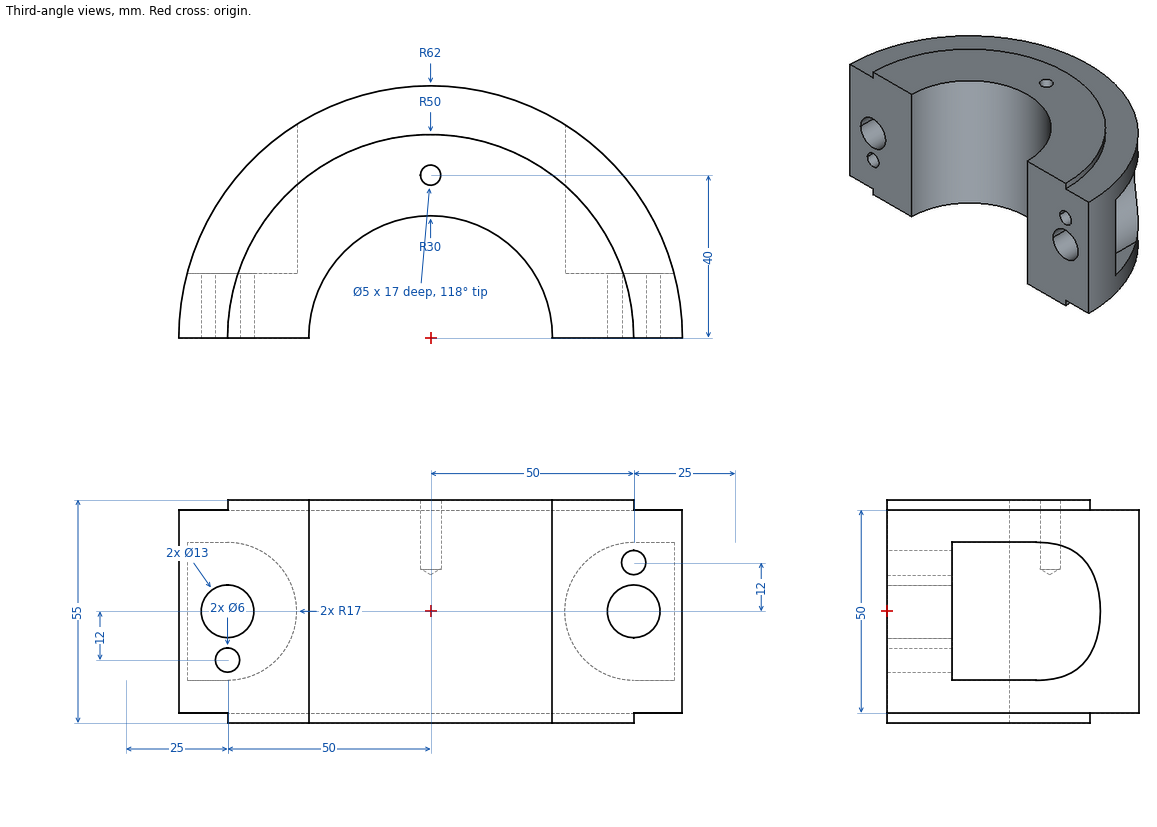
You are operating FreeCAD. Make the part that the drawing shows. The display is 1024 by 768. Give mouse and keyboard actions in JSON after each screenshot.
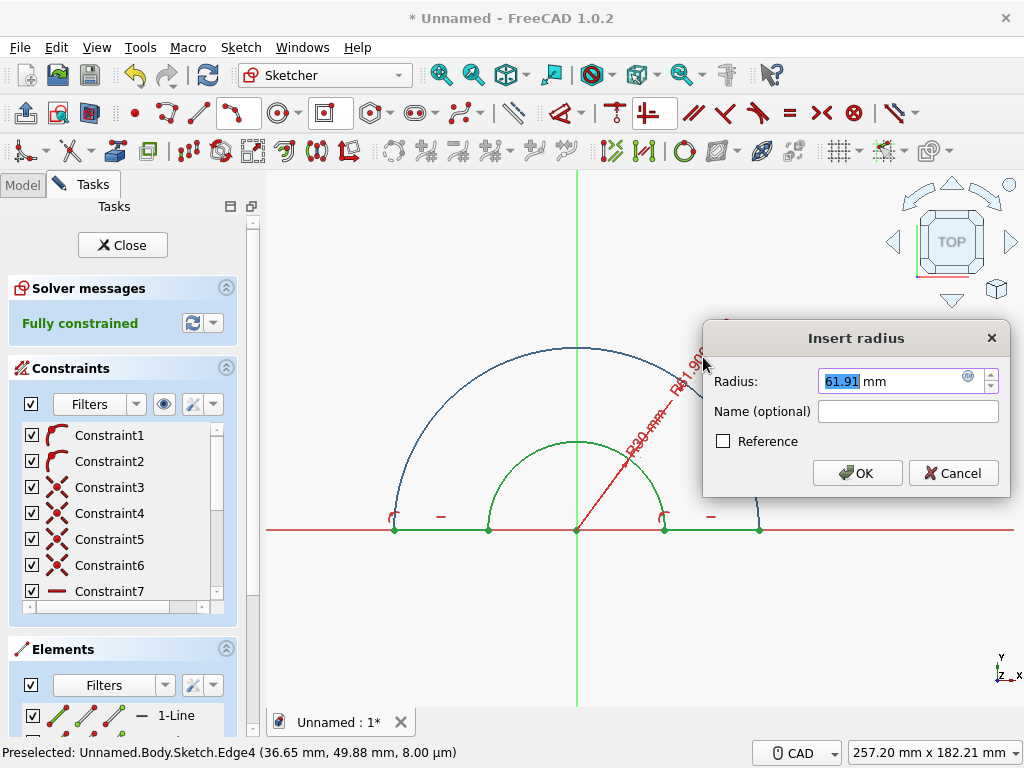
{"action": "type", "text": "62"}
{"action": "key", "text": "Return"}
{"action": "key", "text": "Escape"}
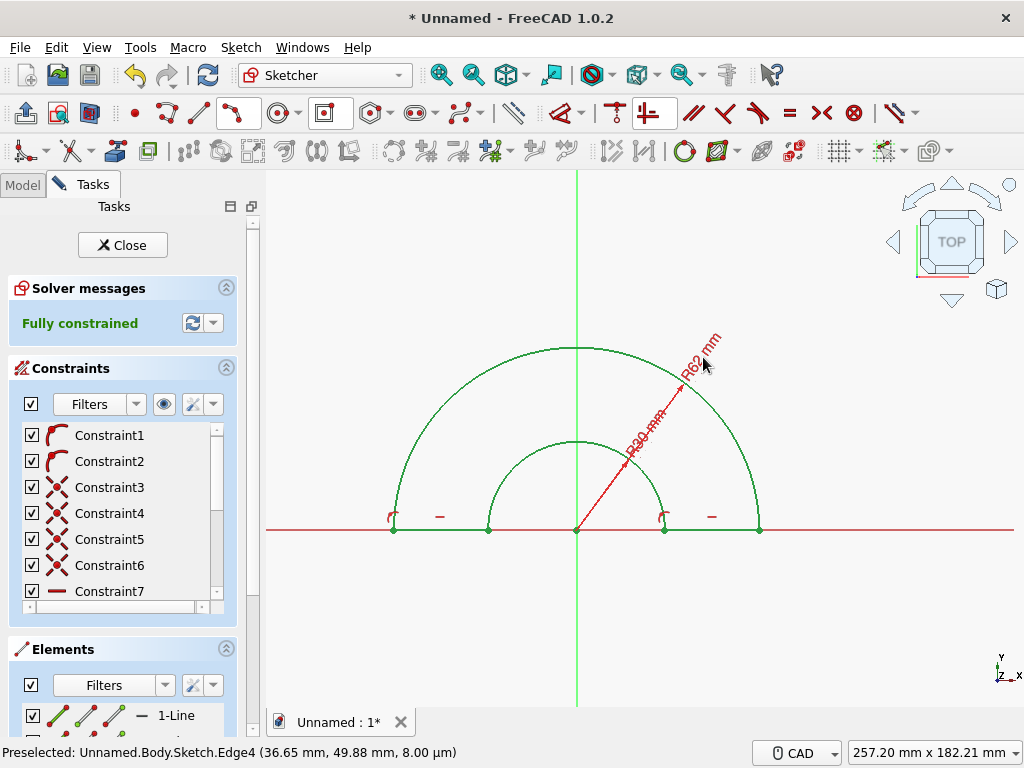
{"action": "left_click", "coordinate": [123, 245]}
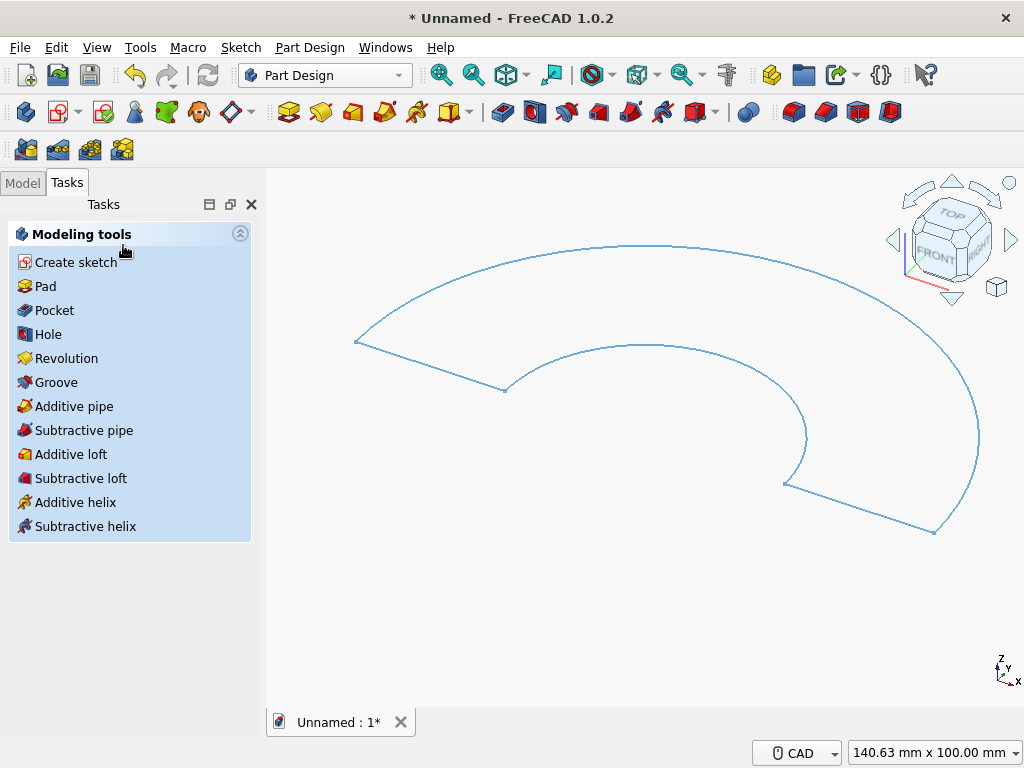
{"action": "left_click", "coordinate": [290, 112]}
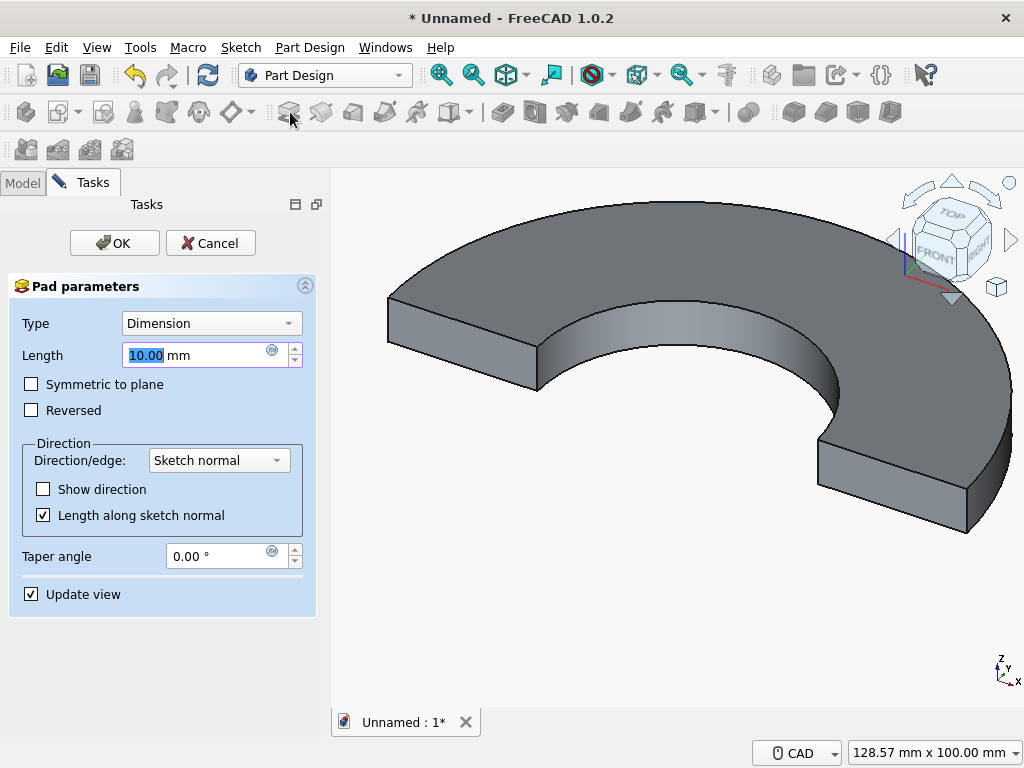
{"action": "type", "text": "50"}
{"action": "key", "text": "Tab"}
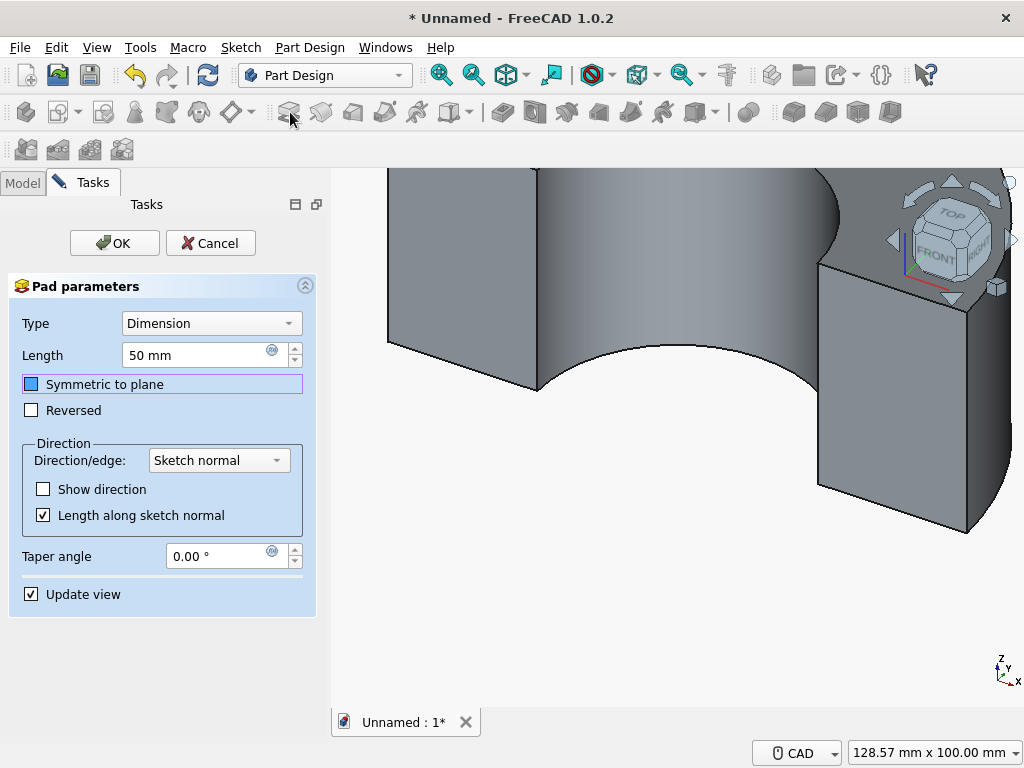
{"action": "left_click", "coordinate": [30, 384]}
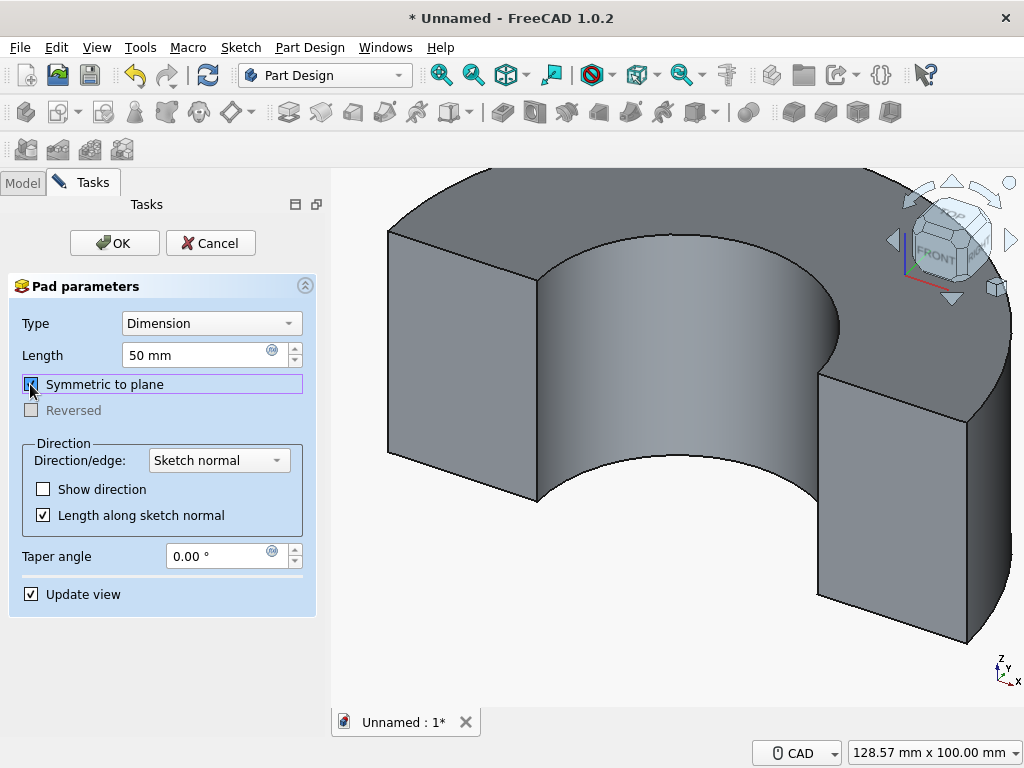
{"action": "left_click", "coordinate": [115, 243]}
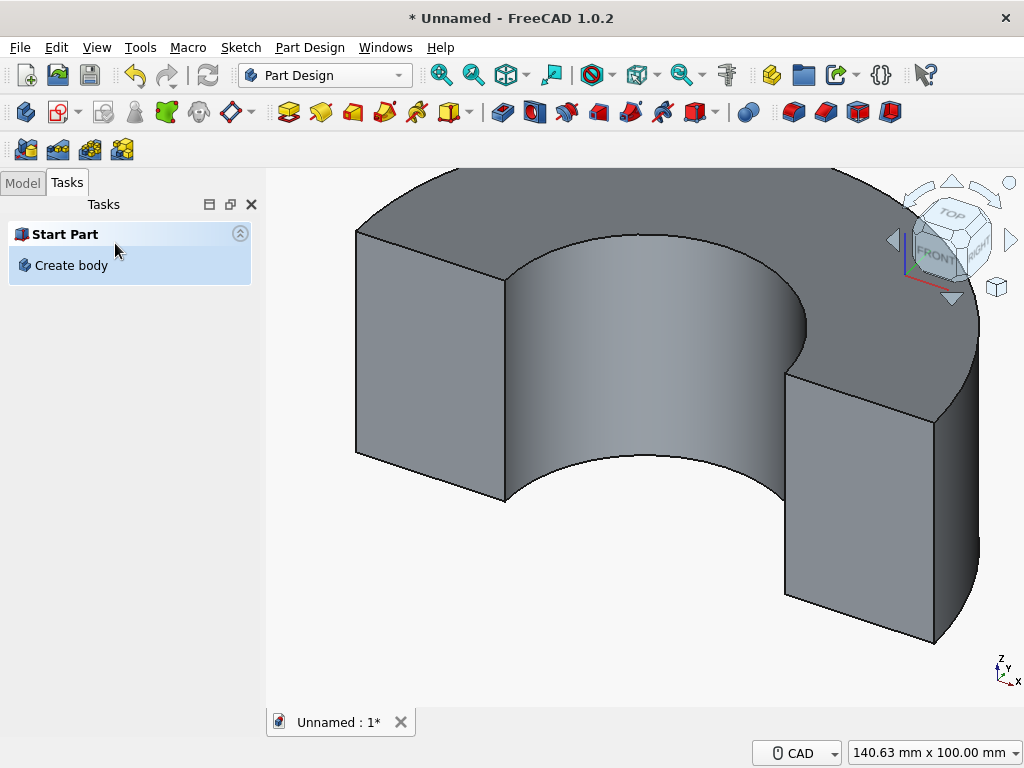
{"action": "left_click", "coordinate": [442, 76]}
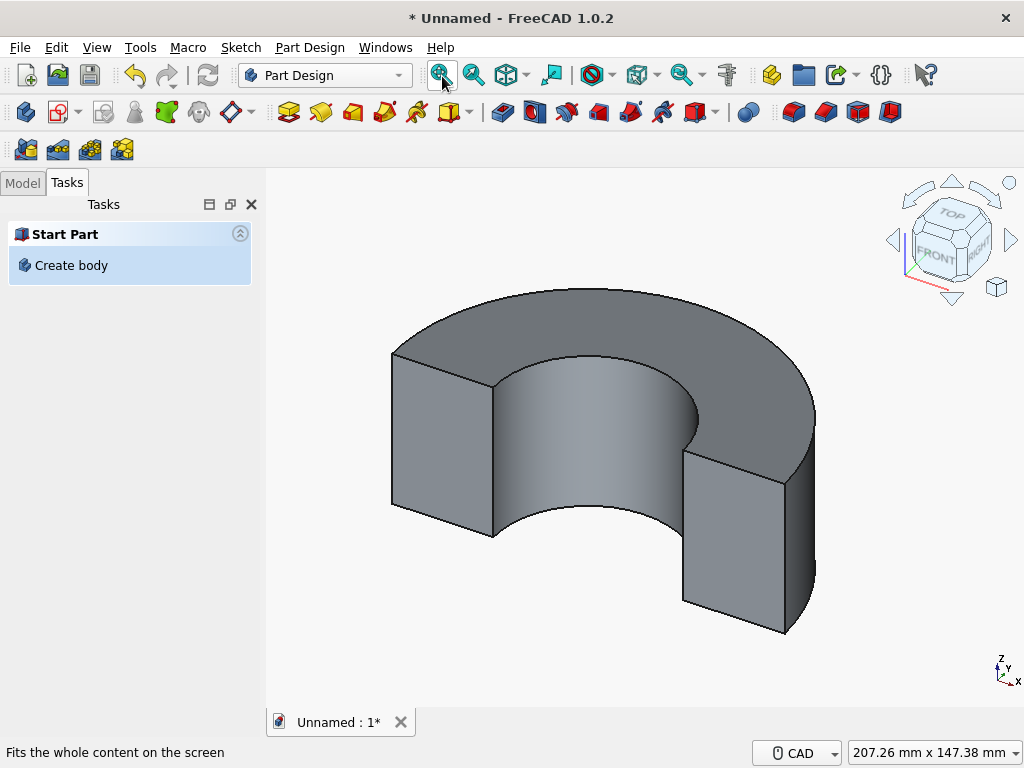
{"action": "left_click", "coordinate": [58, 112]}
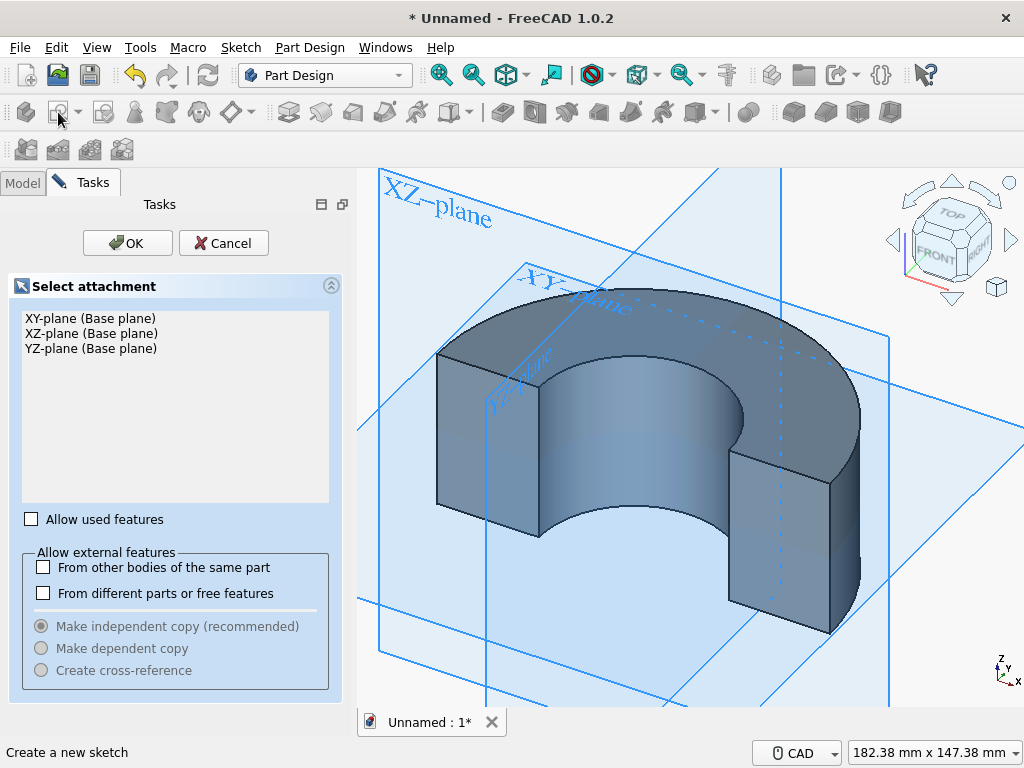
{"action": "left_click", "coordinate": [82, 318]}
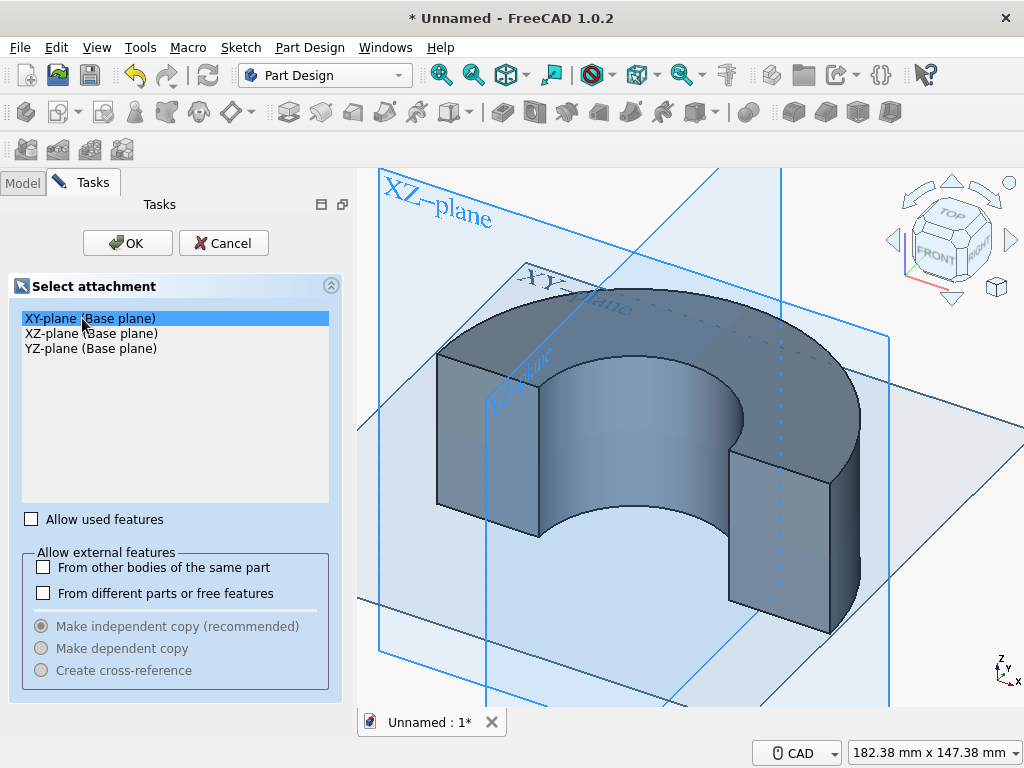
{"action": "left_click", "coordinate": [128, 243]}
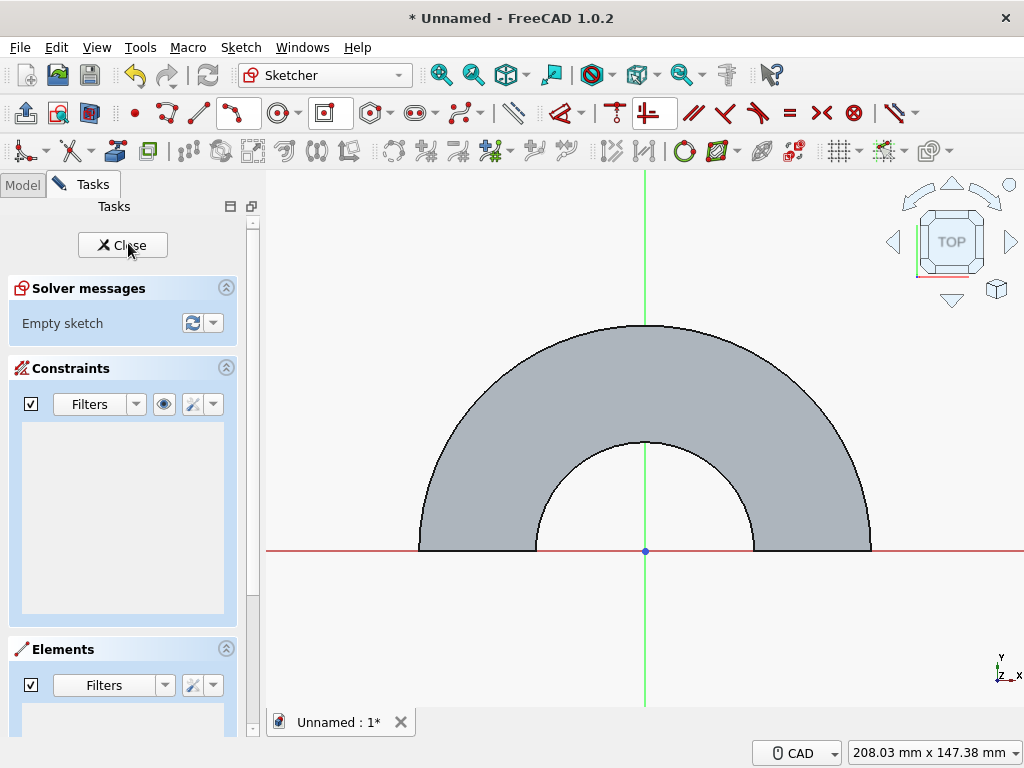
{"action": "left_click", "coordinate": [90, 114]}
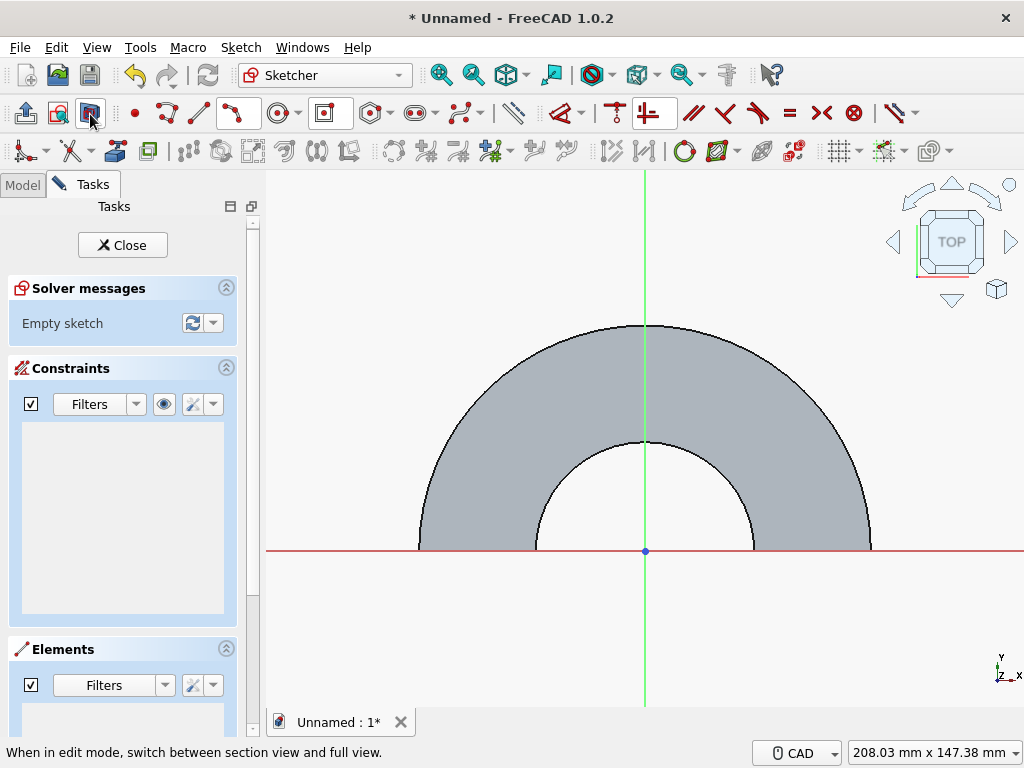
{"action": "left_click", "coordinate": [200, 114]}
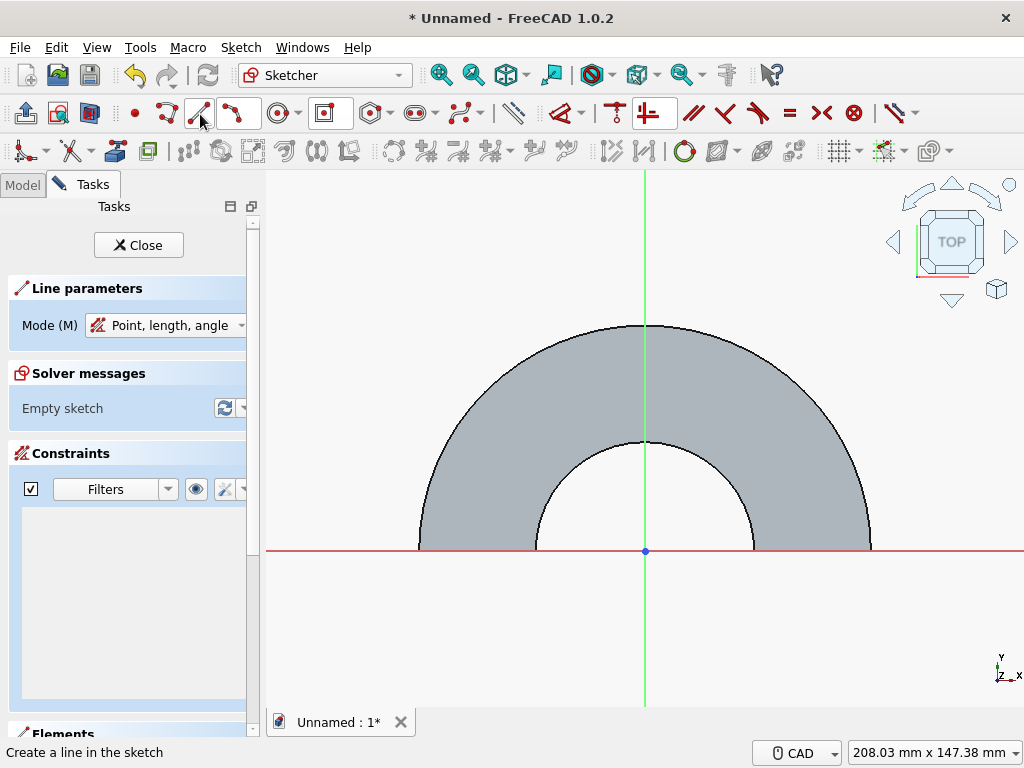
{"action": "left_click", "coordinate": [463, 551]}
{"action": "left_click", "coordinate": [536, 542]}